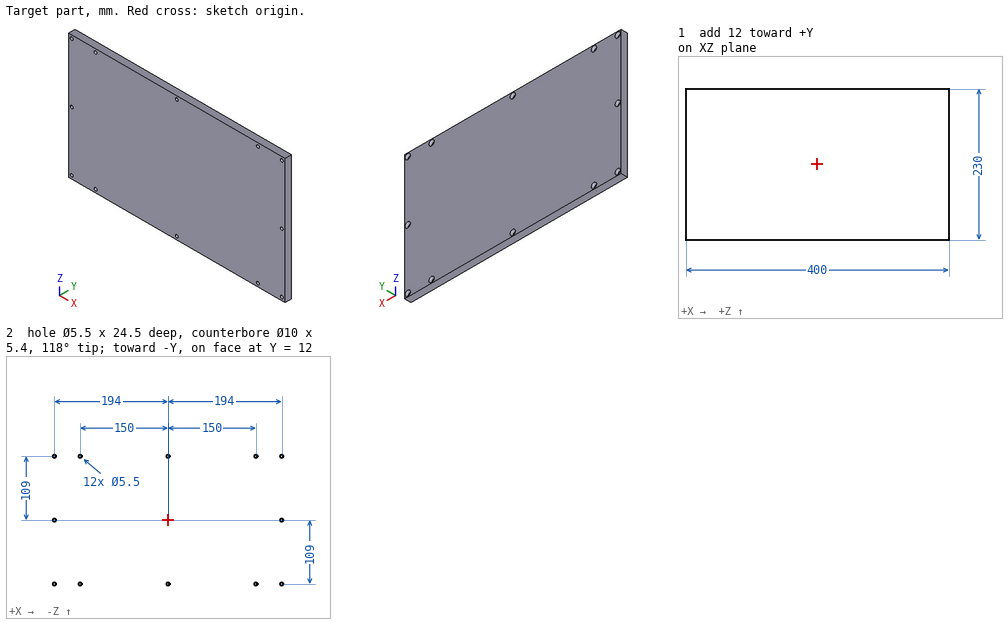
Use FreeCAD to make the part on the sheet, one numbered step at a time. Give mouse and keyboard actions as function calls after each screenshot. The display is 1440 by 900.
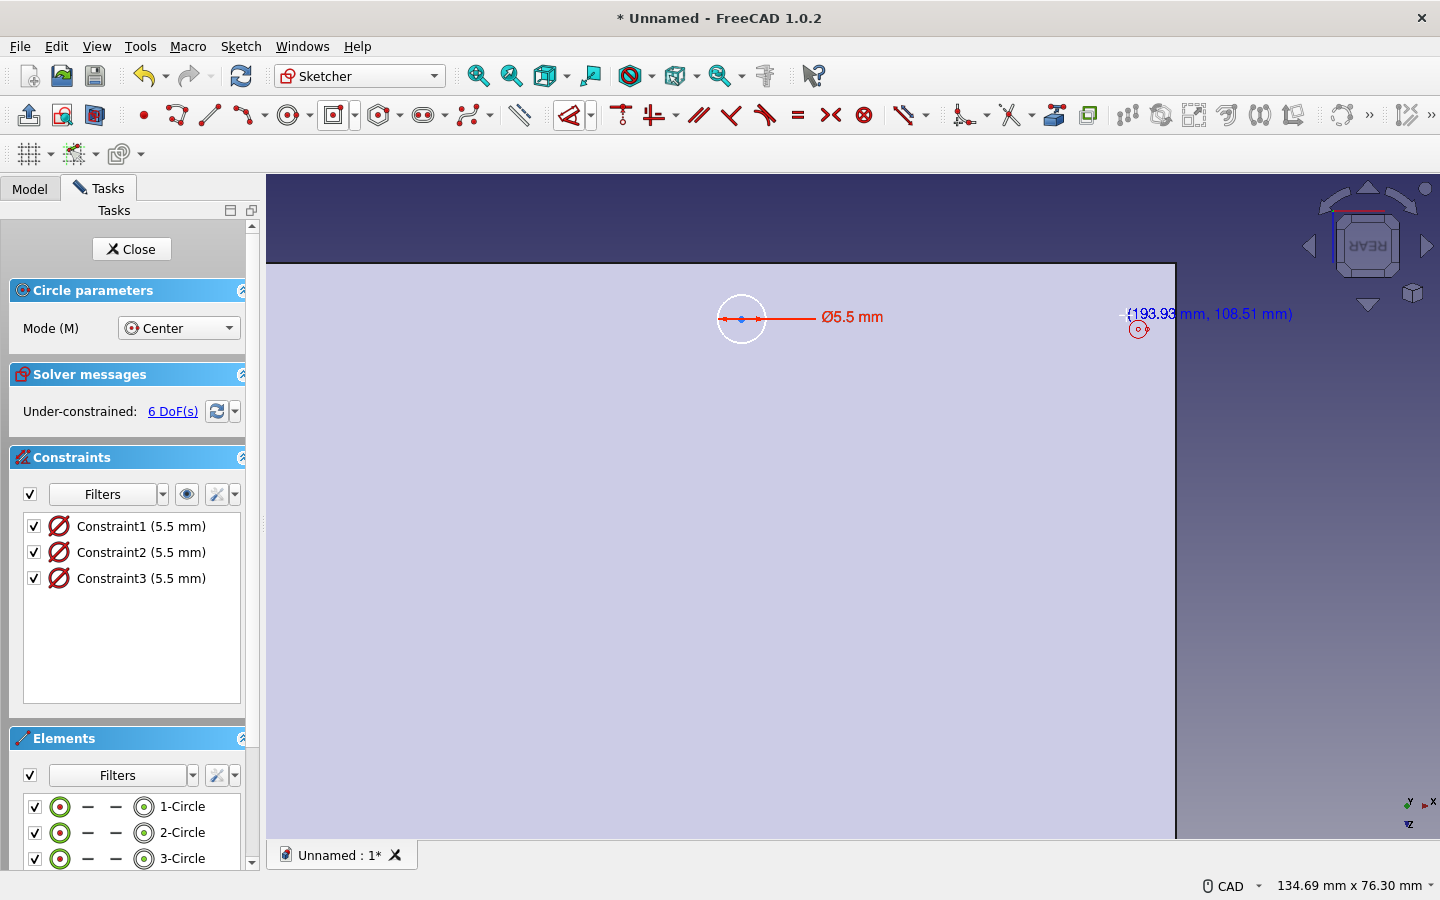
scroll(1126, 315, down, 8)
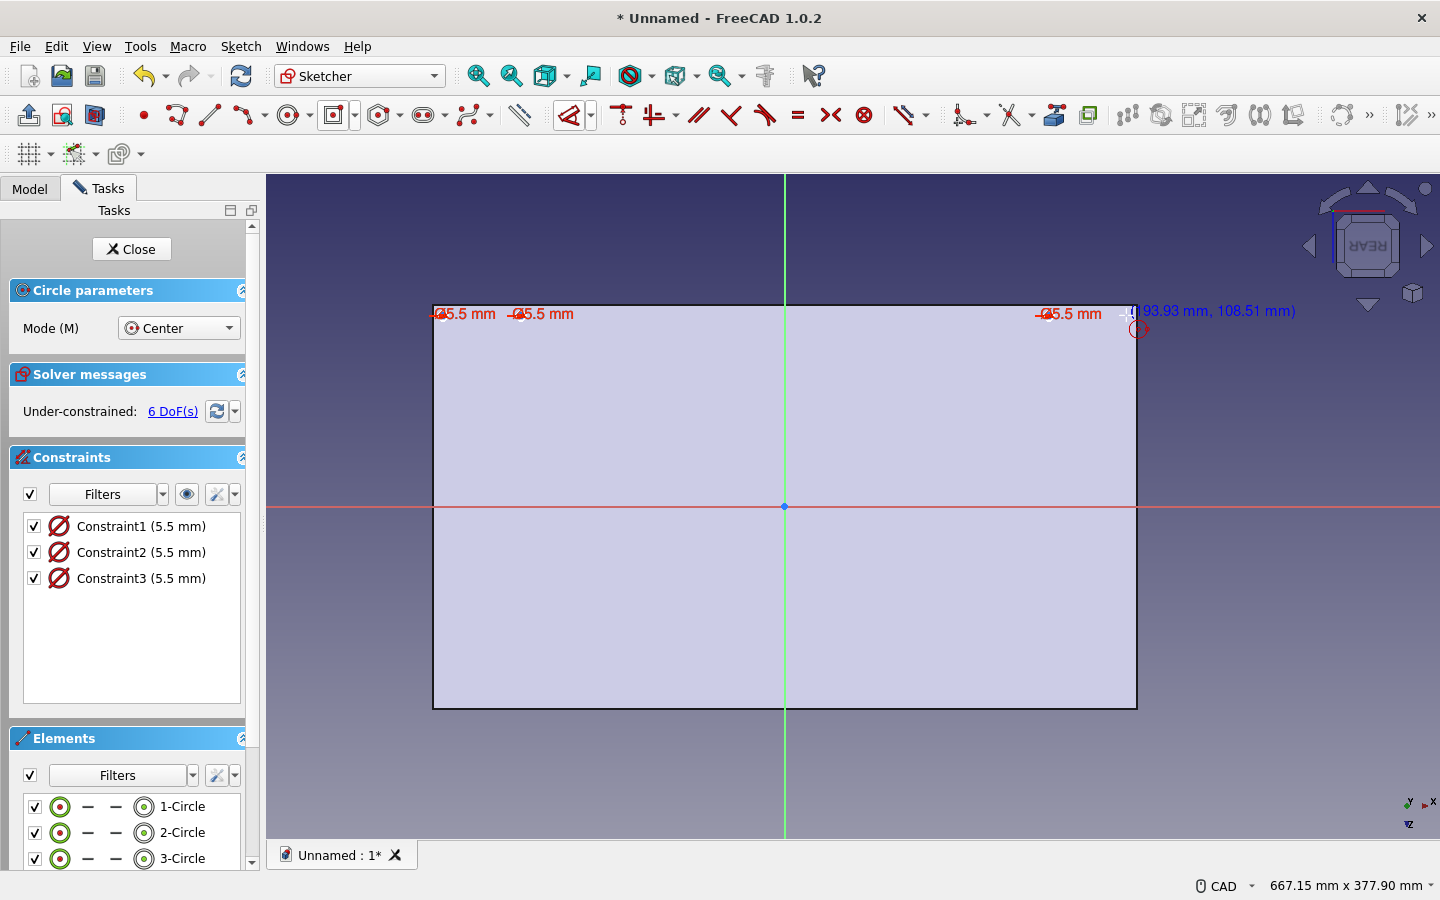
click(1126, 315)
move(1130, 312)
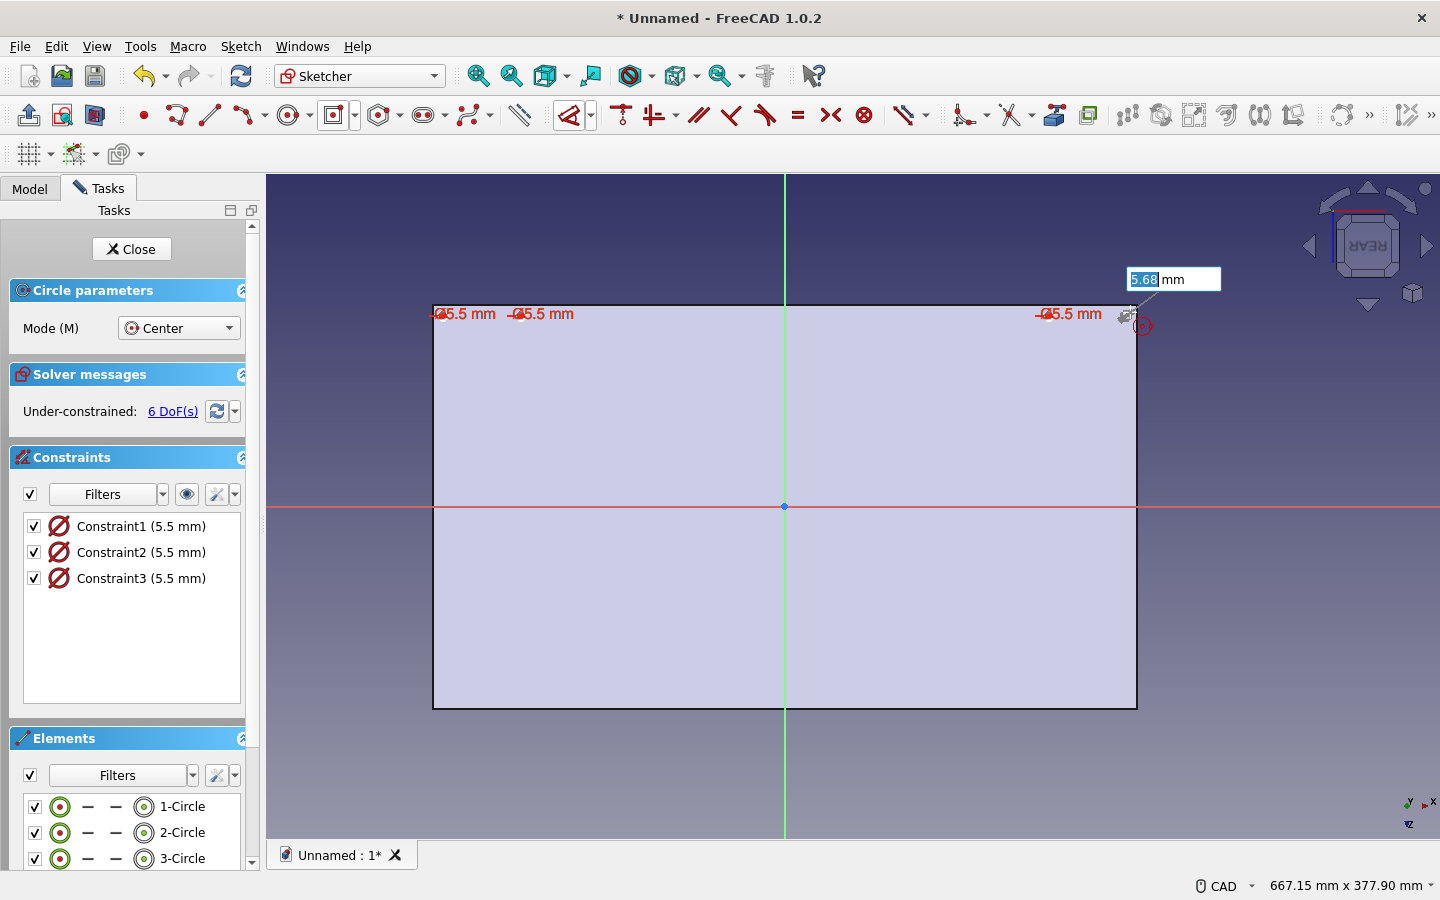
text(5.5)
key(Return)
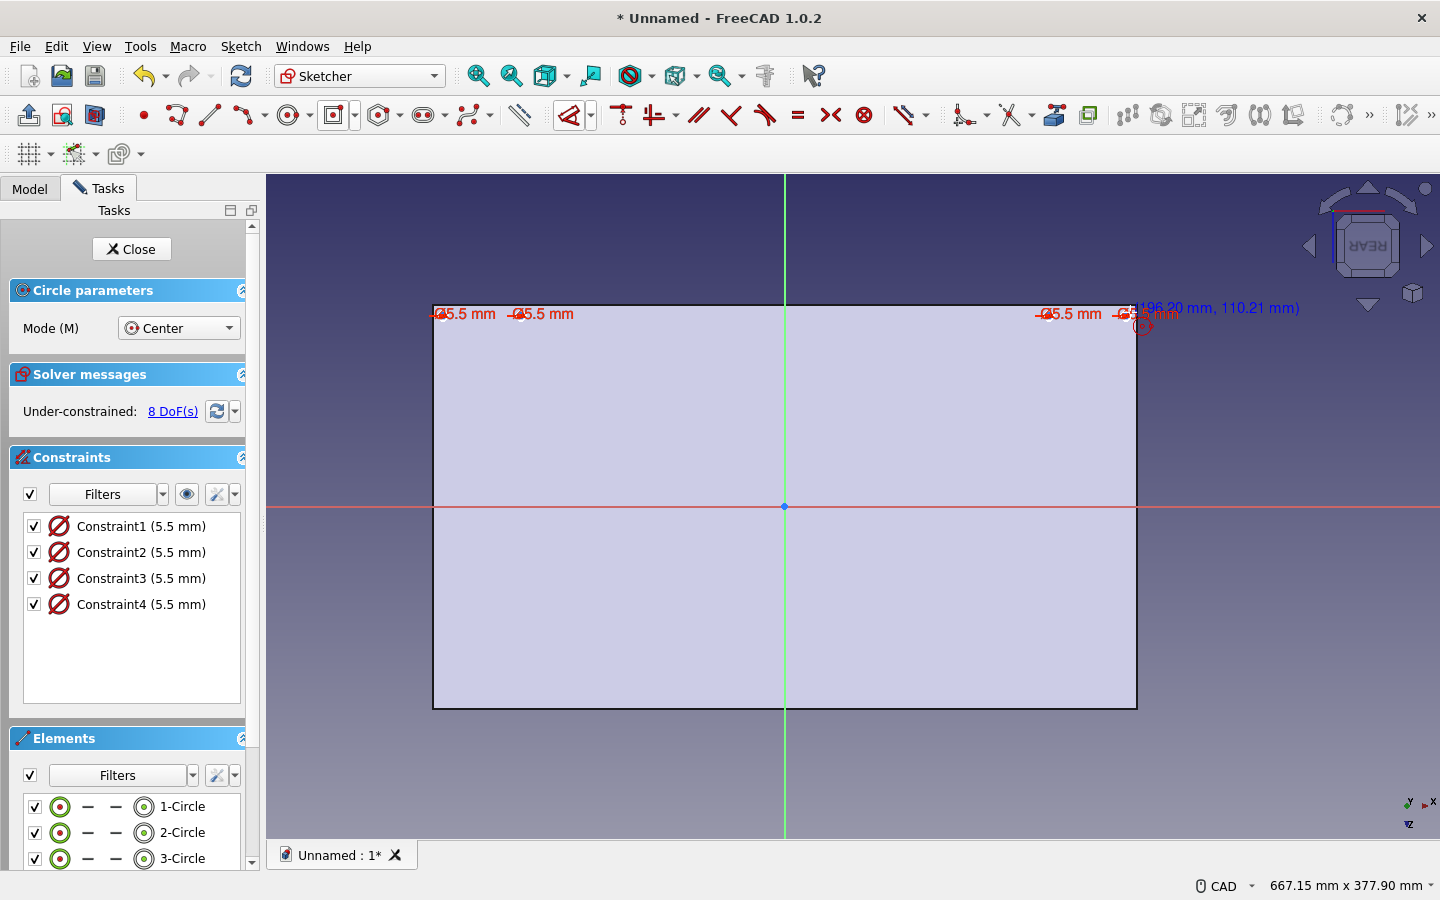
scroll(1126, 507, up, 8)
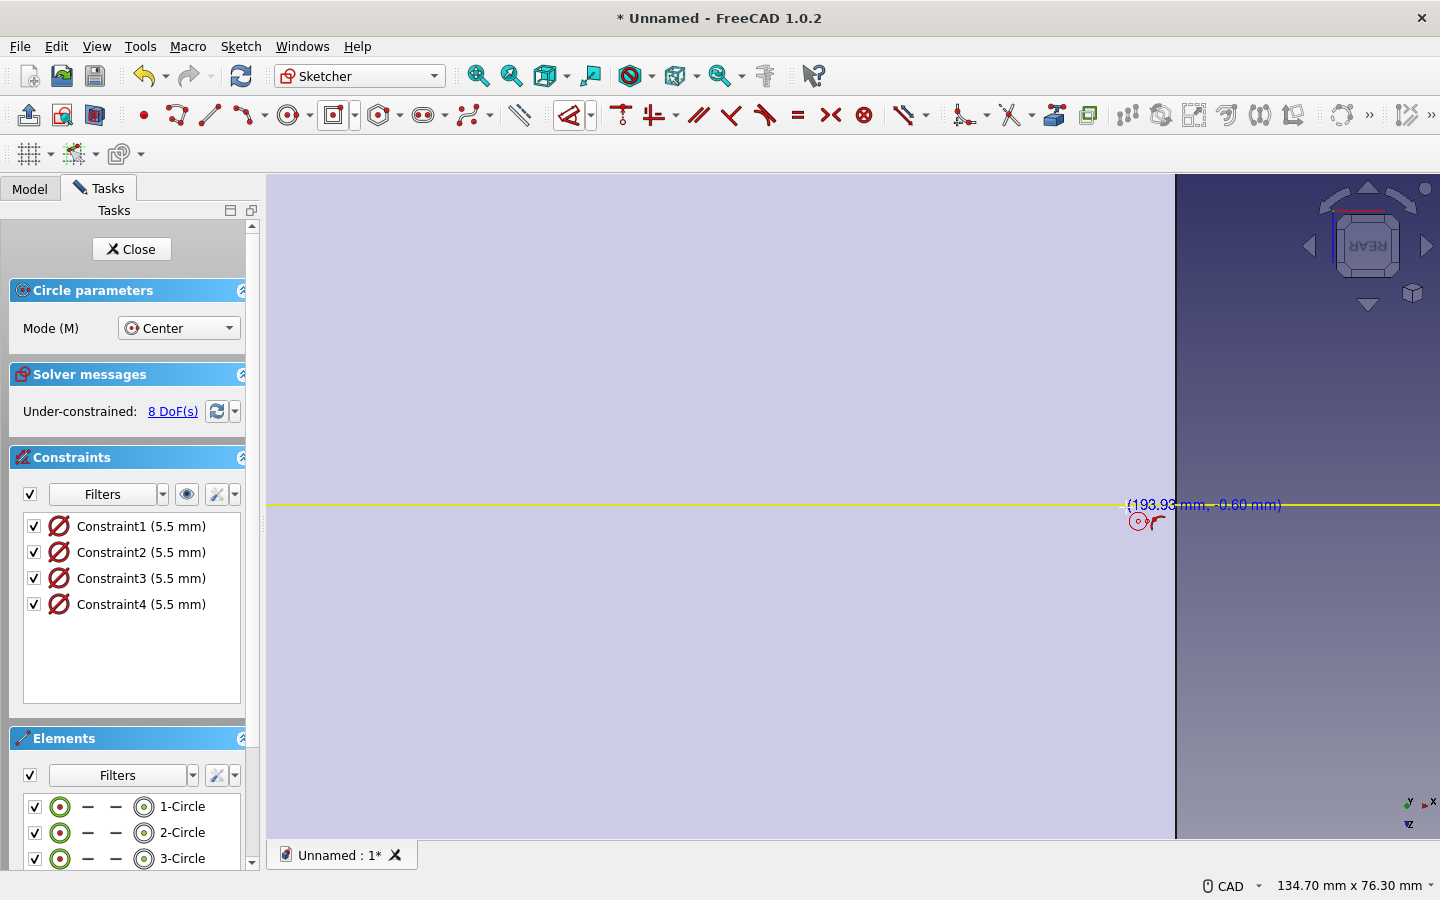
scroll(1126, 507, down, 8)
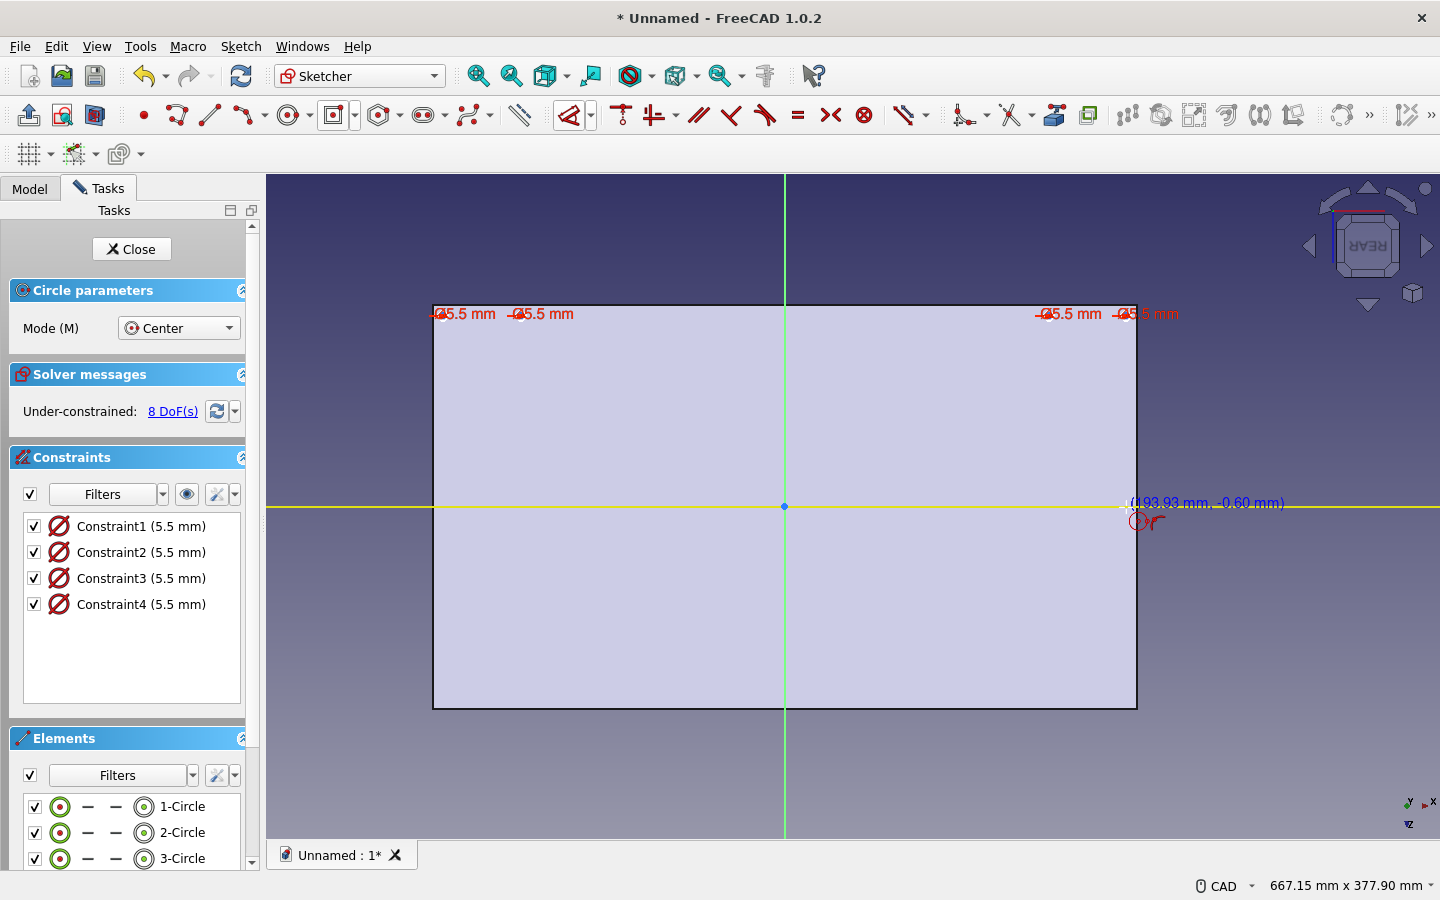
click(1126, 507)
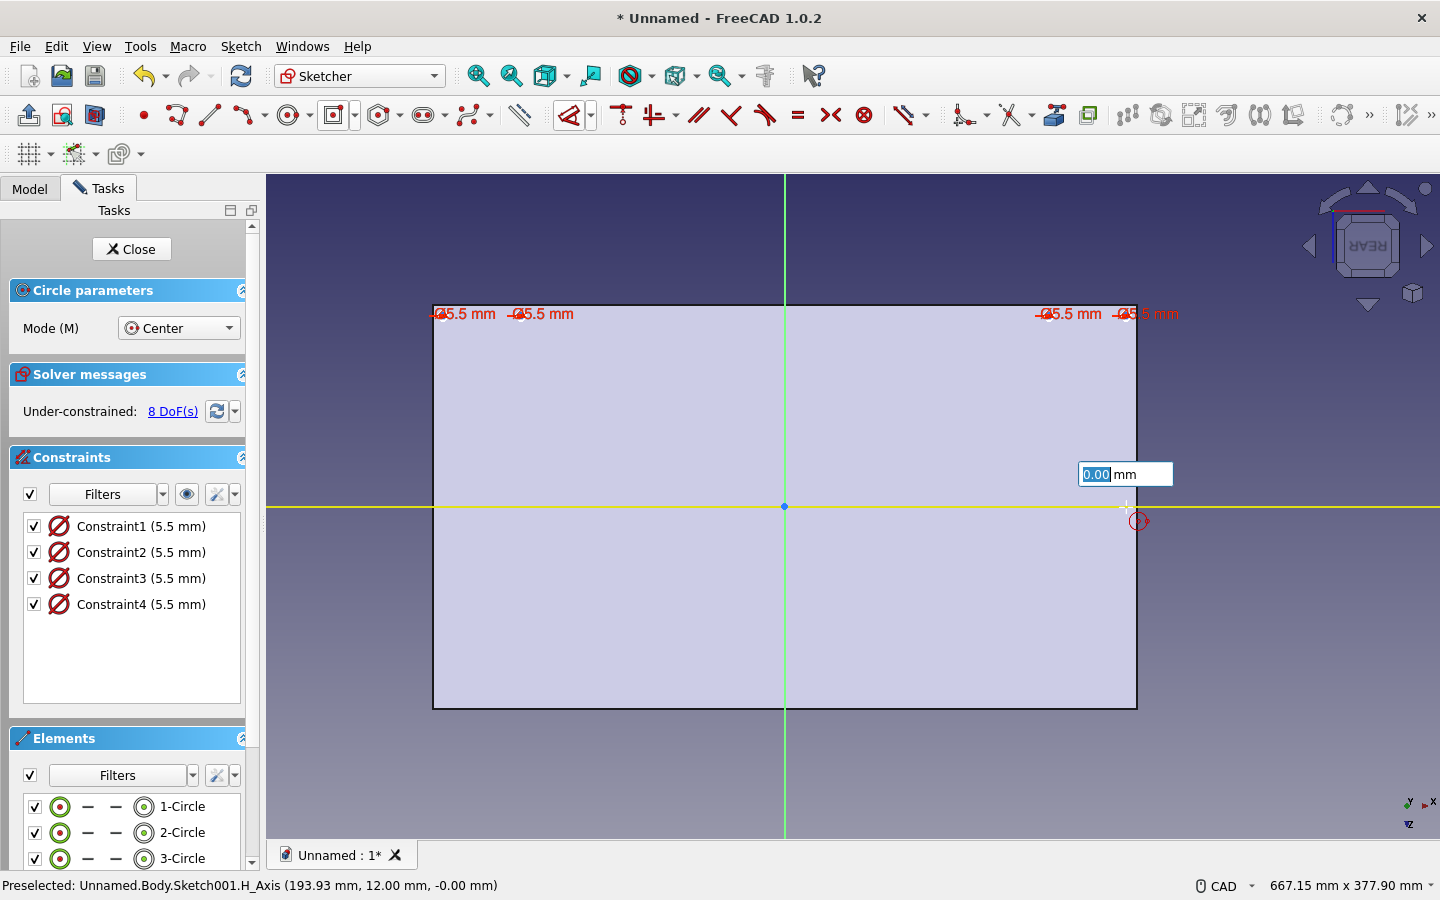
scroll(1128, 502, up, 7)
move(1125, 502)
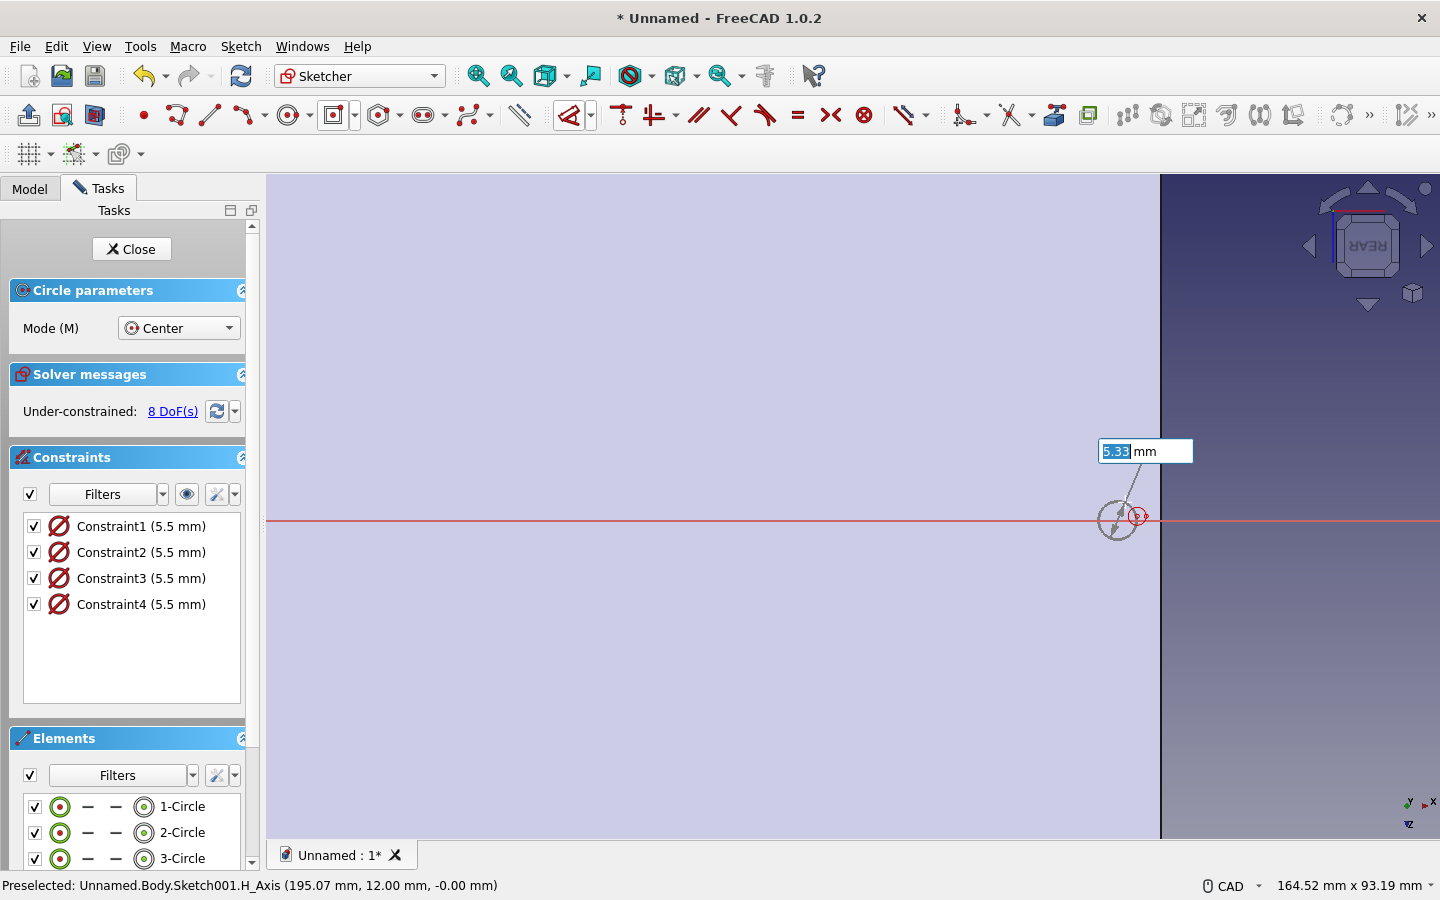
text(5.5)
key(Return)